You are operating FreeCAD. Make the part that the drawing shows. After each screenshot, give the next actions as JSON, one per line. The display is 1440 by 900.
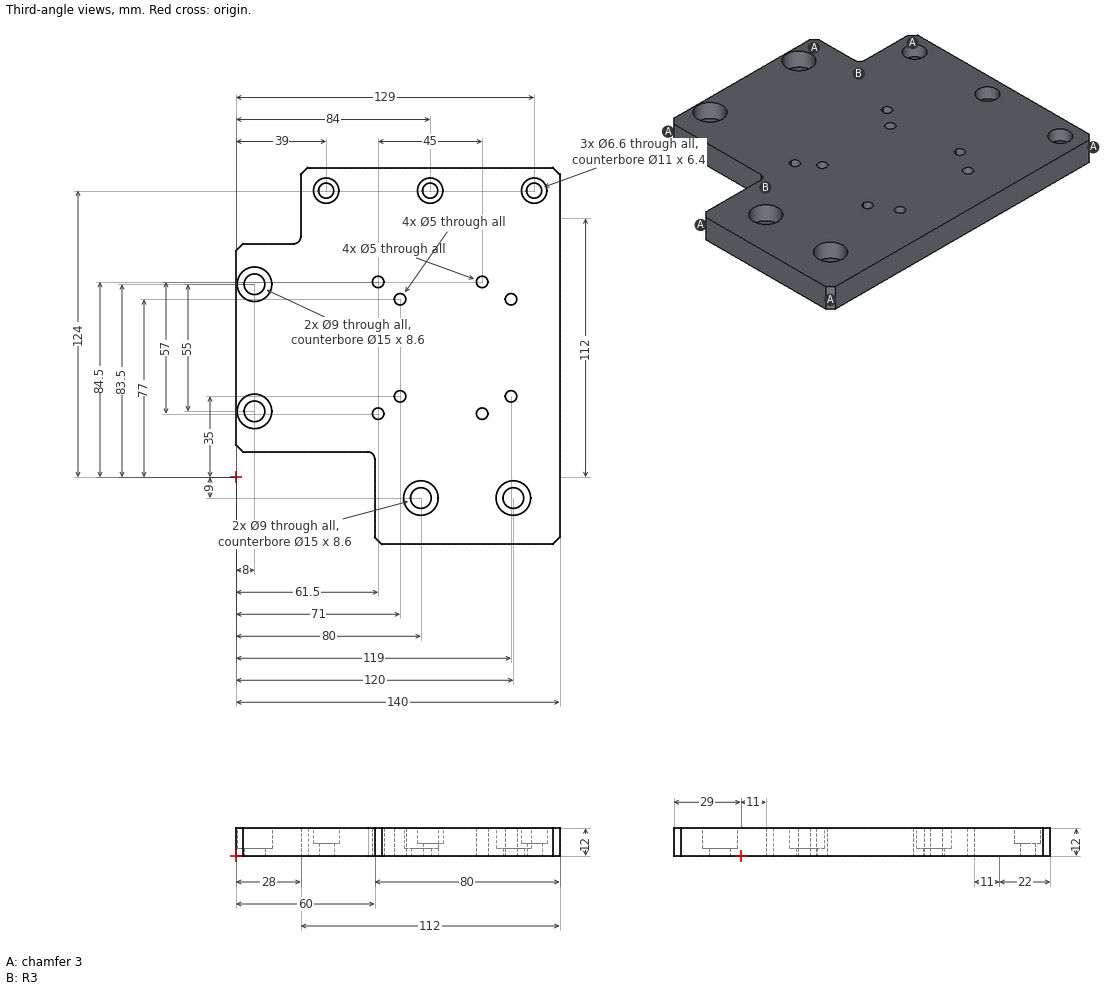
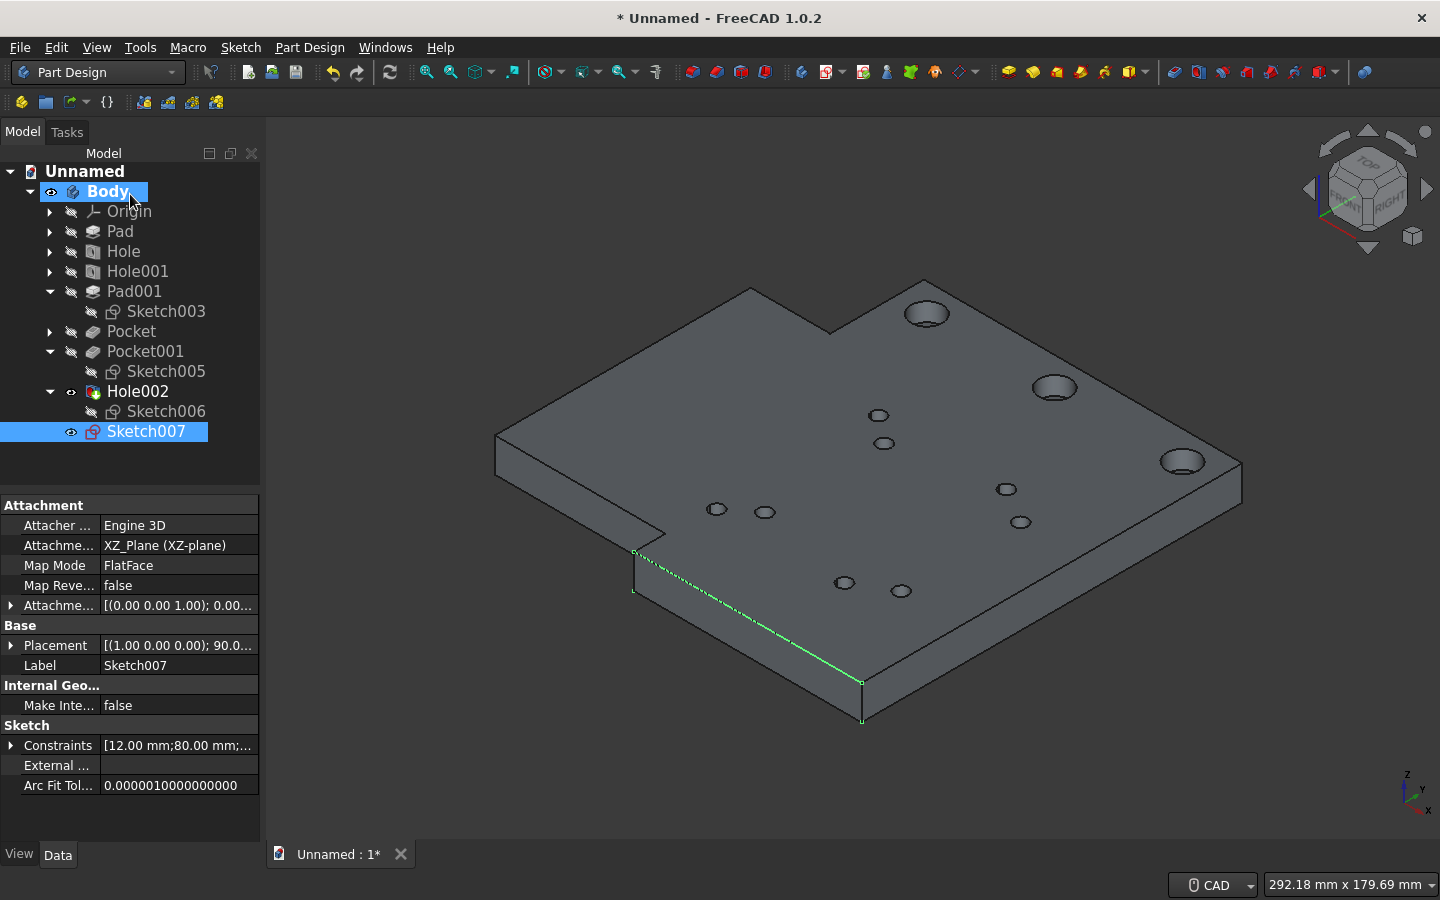
{"action": "left_click", "coordinate": [1010, 72]}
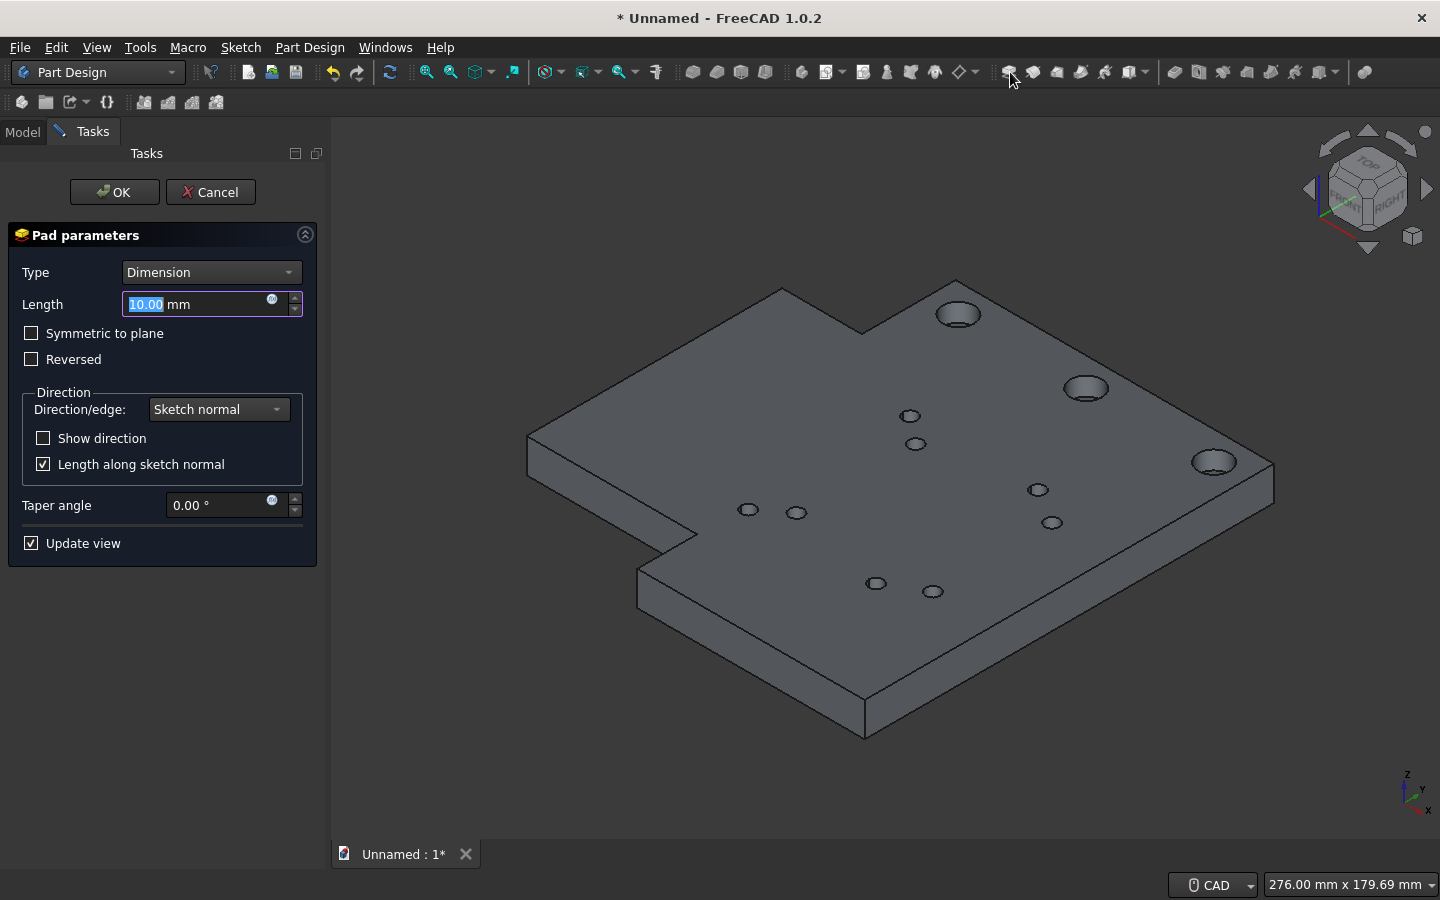
{"action": "type", "text": "29"}
{"action": "key", "text": "Tab"}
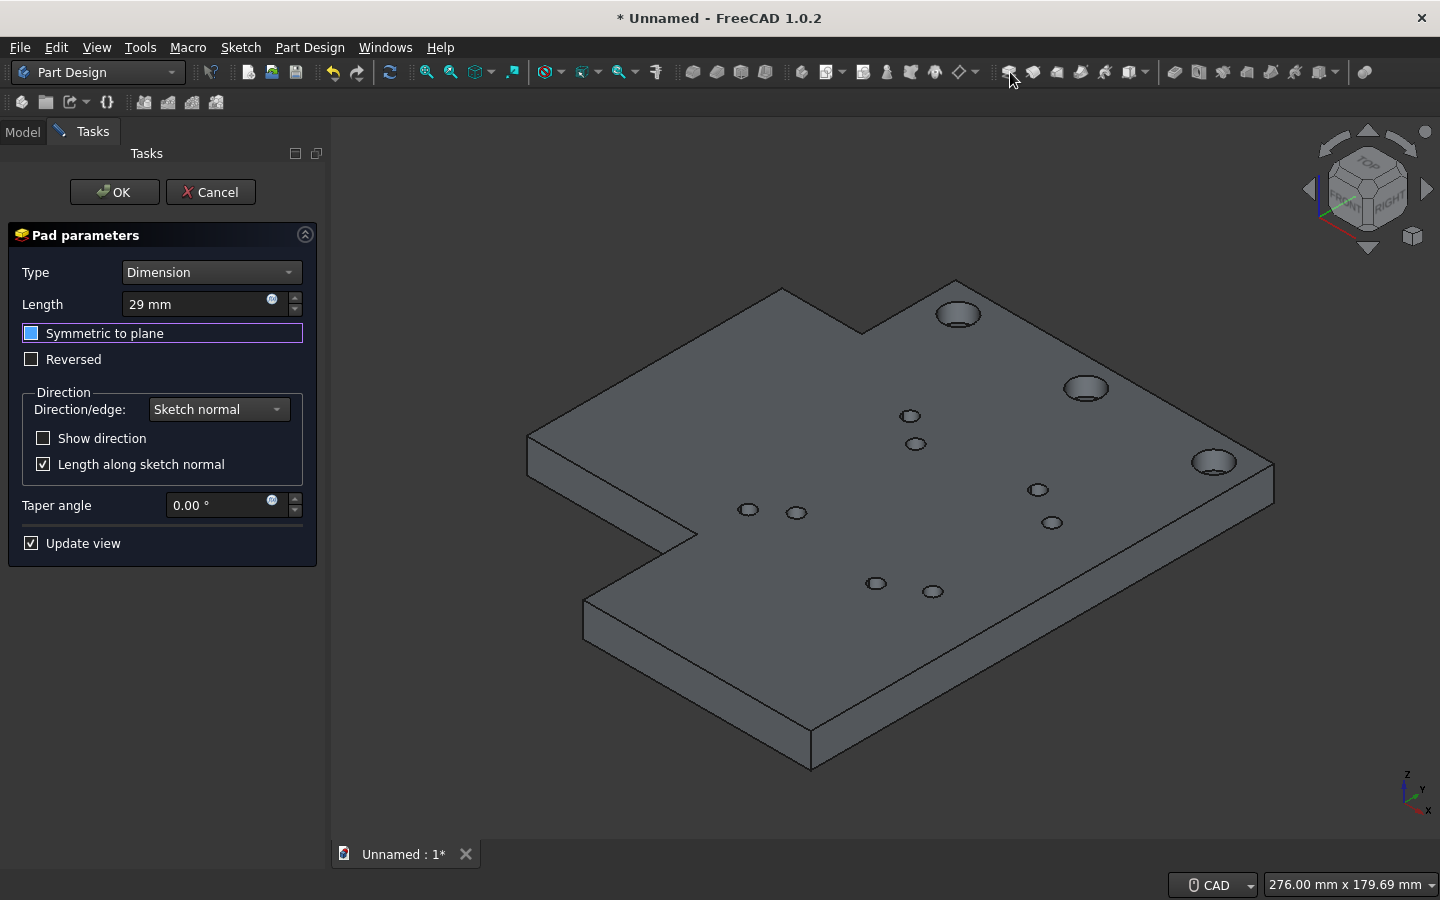
{"action": "left_click", "coordinate": [115, 192]}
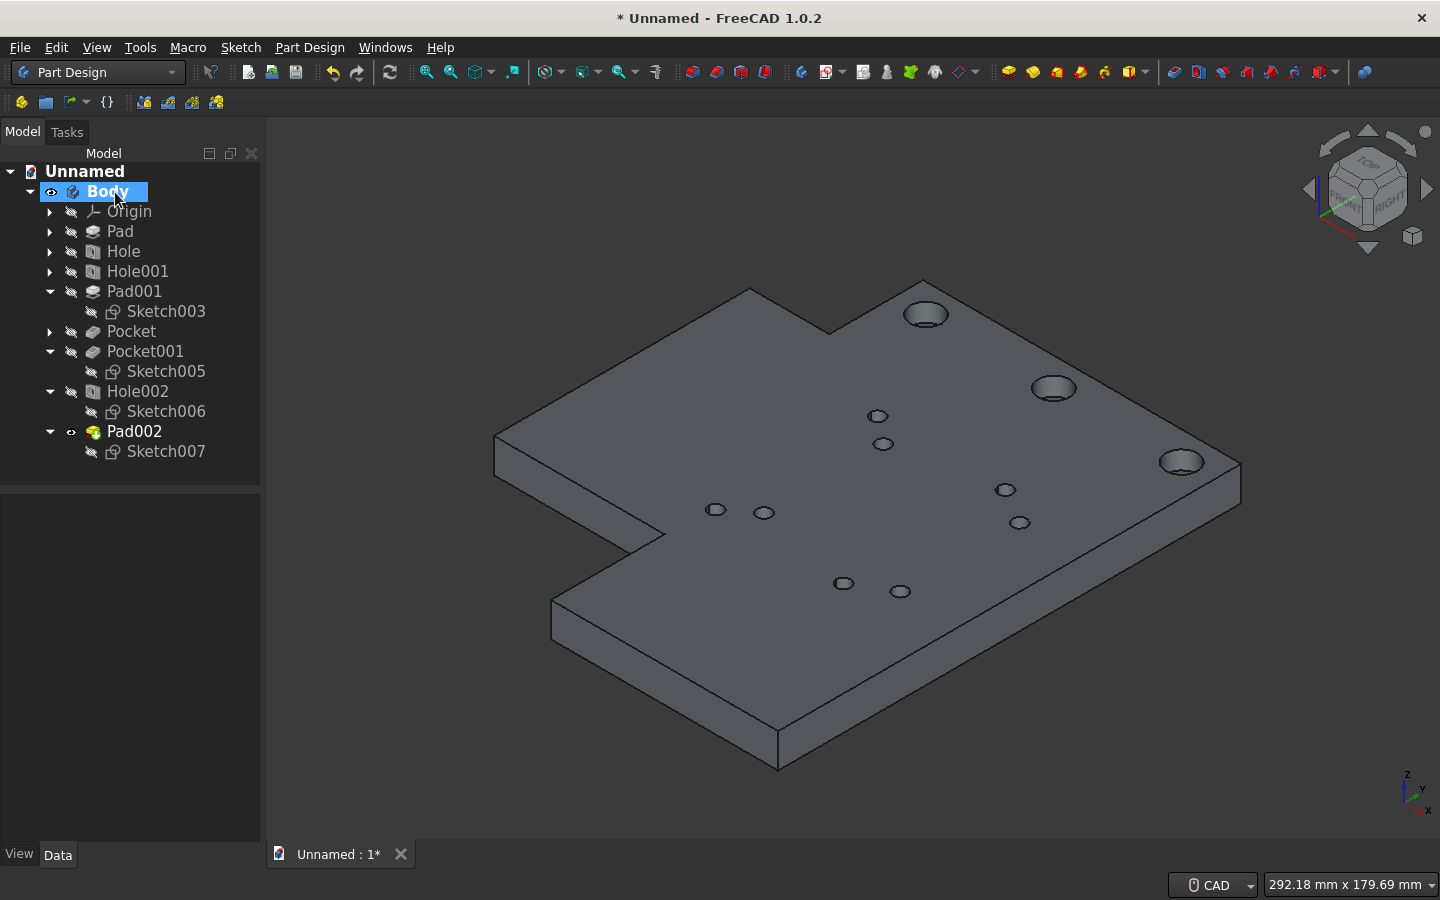
{"action": "left_click", "coordinate": [778, 750]}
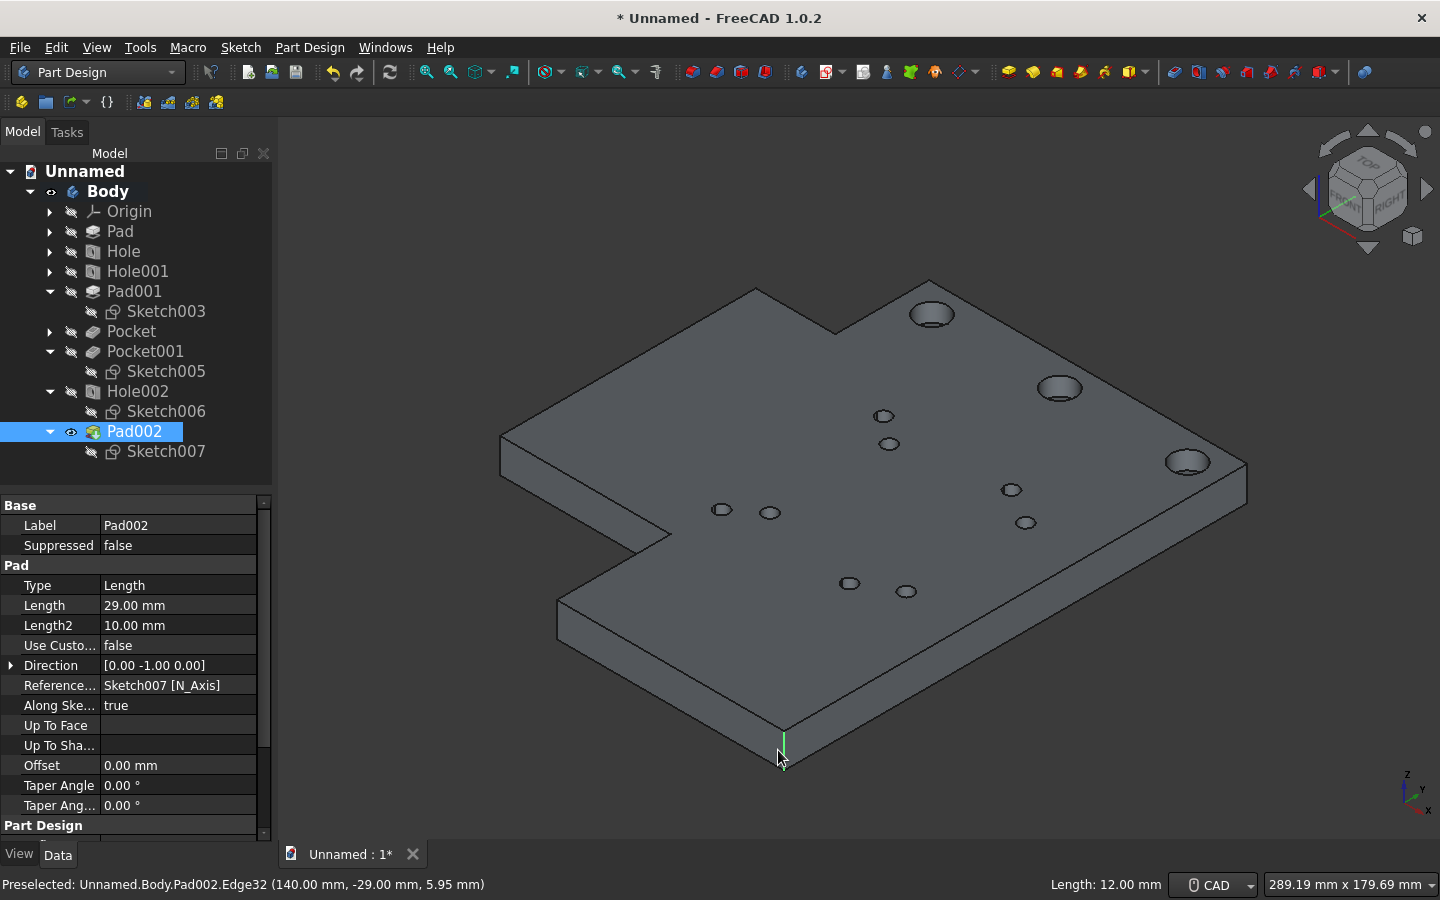
{"action": "key", "text": "2"}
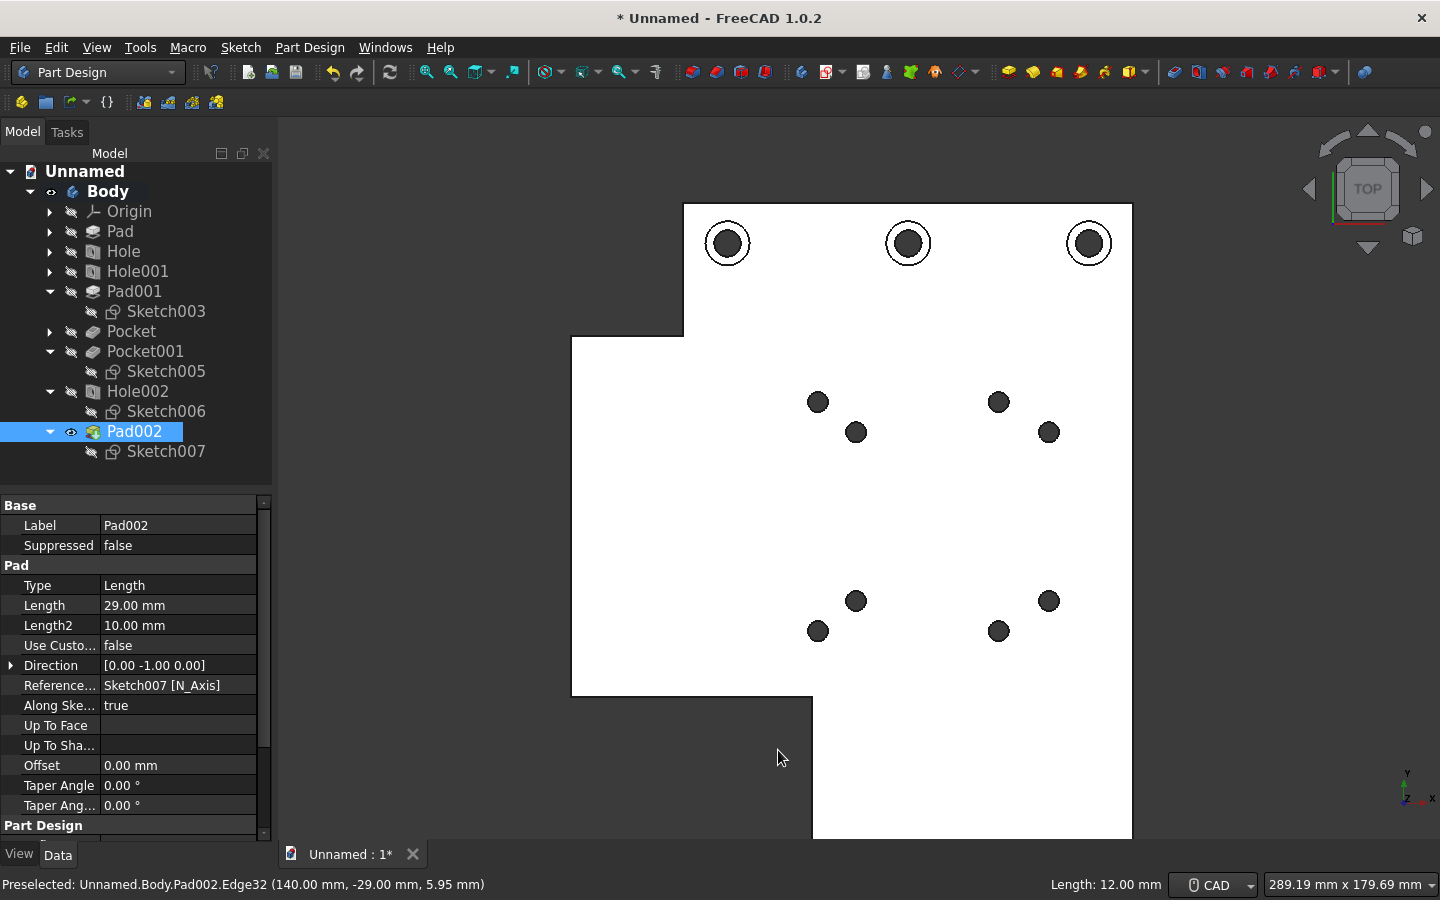
{"action": "key", "text": "v f"}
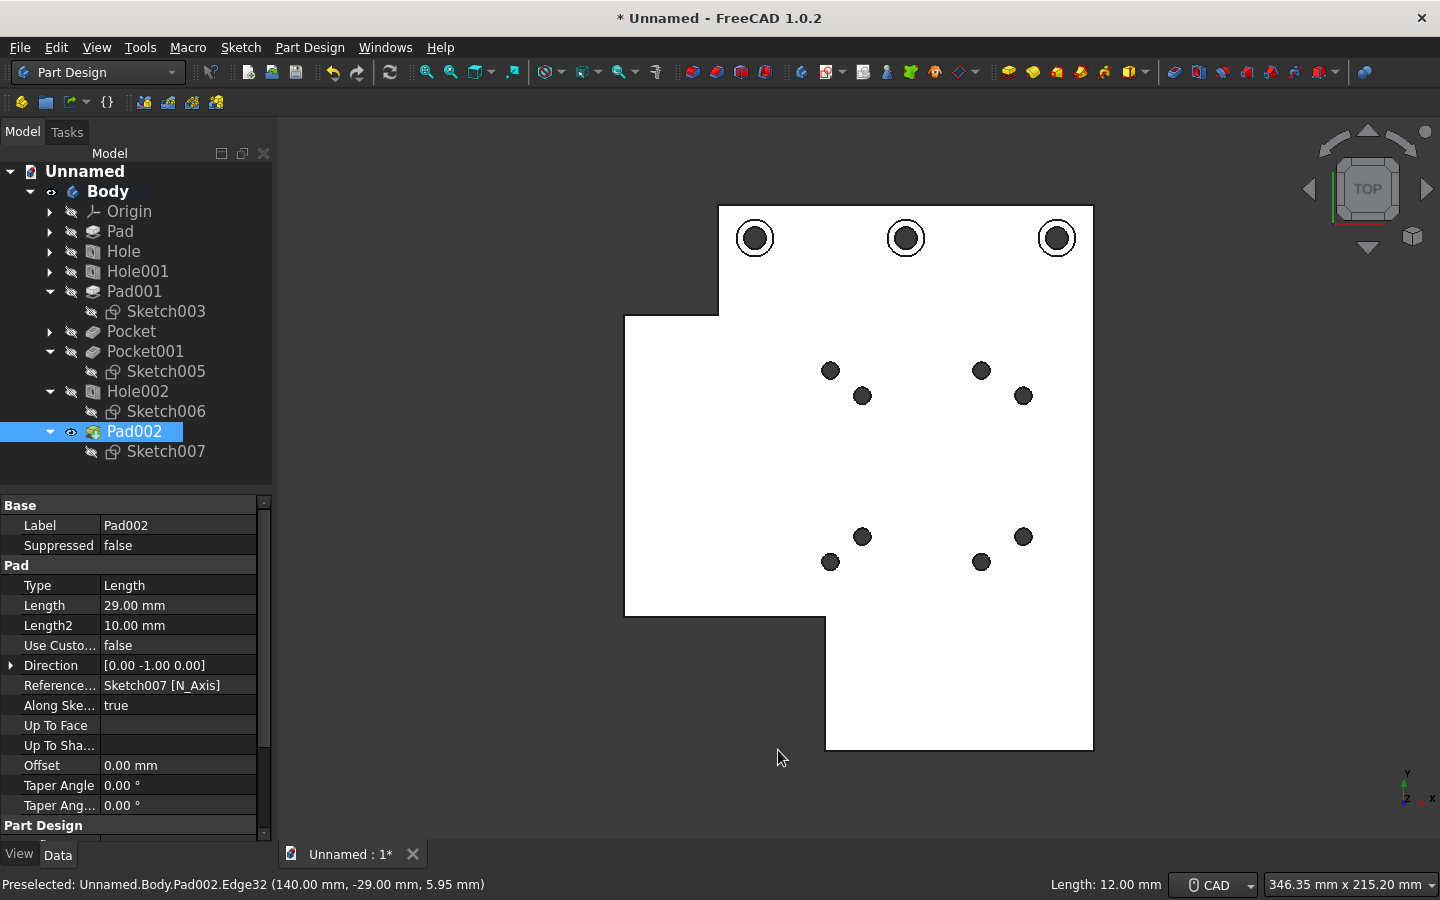
{"action": "key", "text": "0"}